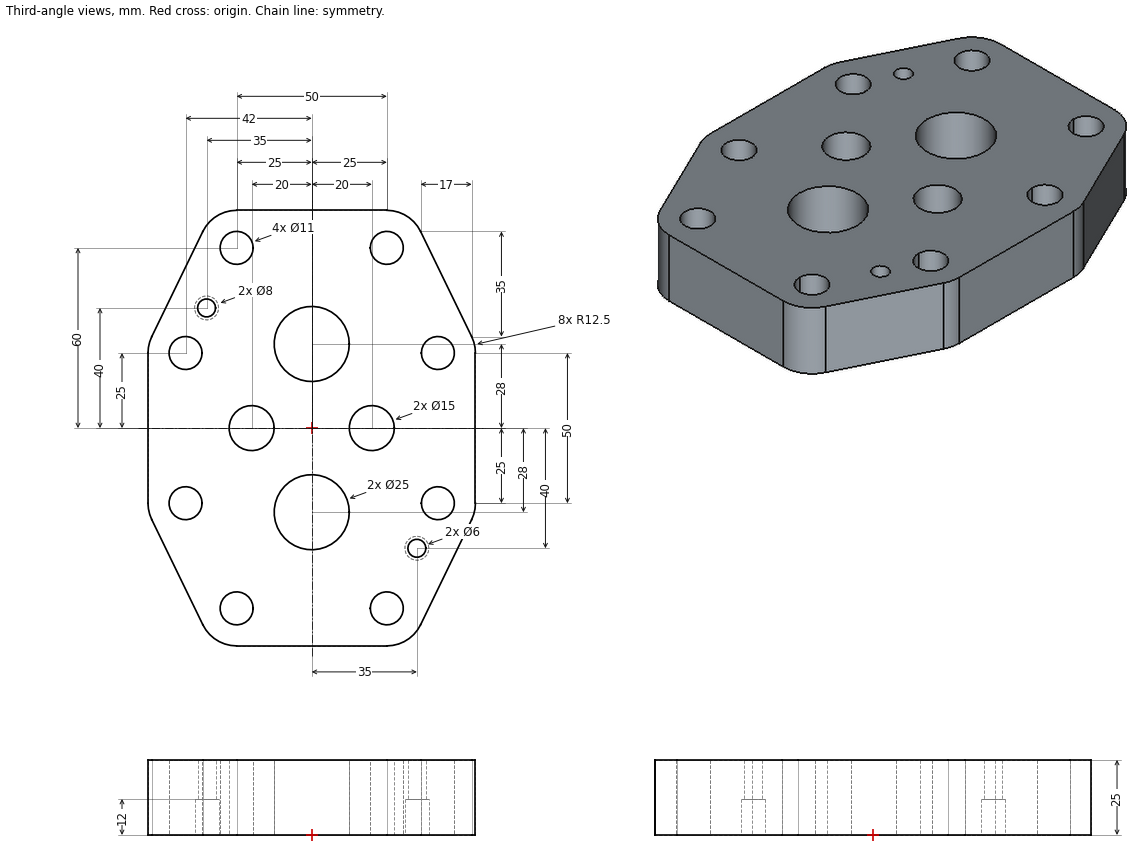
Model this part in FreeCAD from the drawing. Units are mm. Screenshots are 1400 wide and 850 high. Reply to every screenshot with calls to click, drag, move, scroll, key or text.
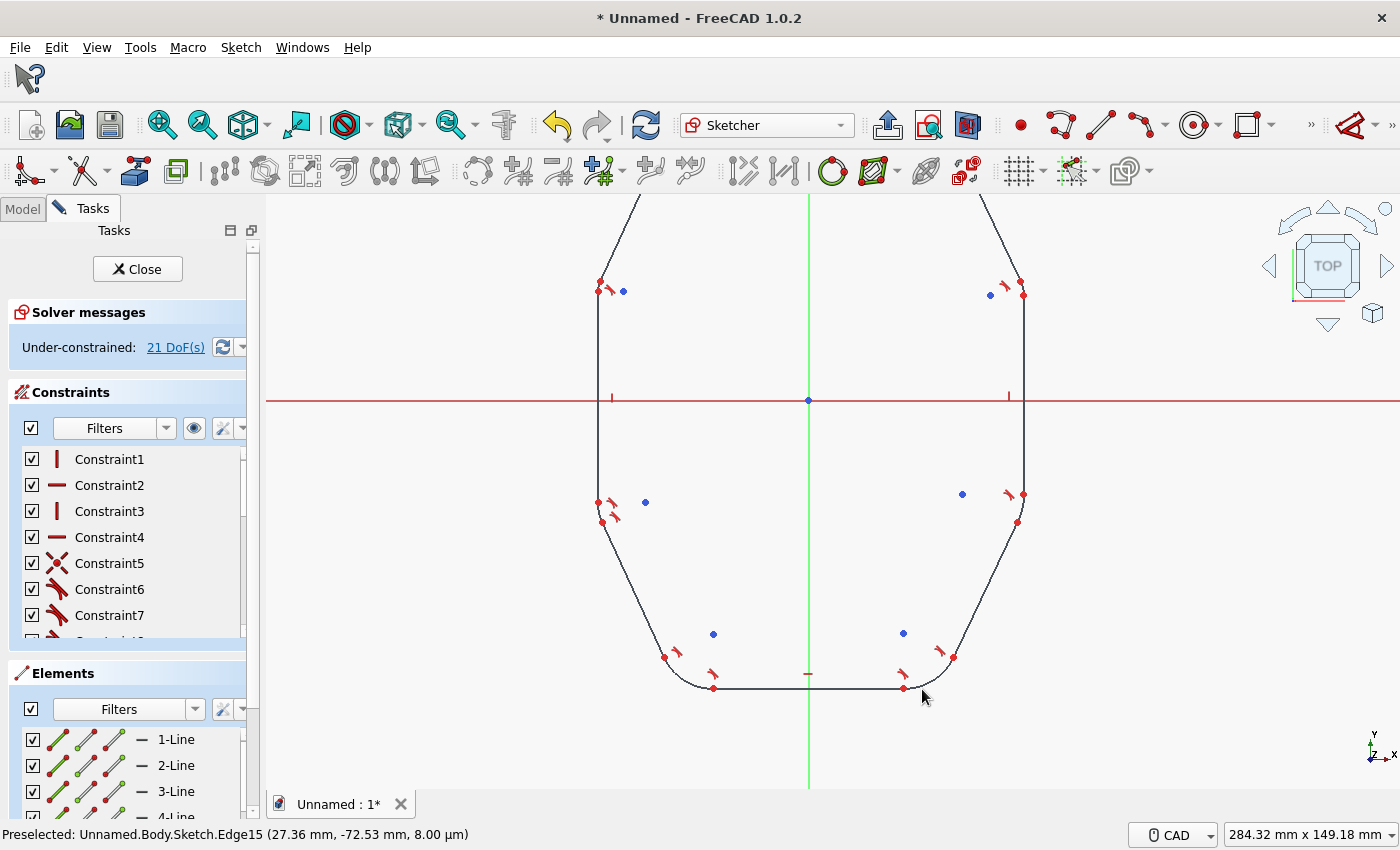
click(973, 617)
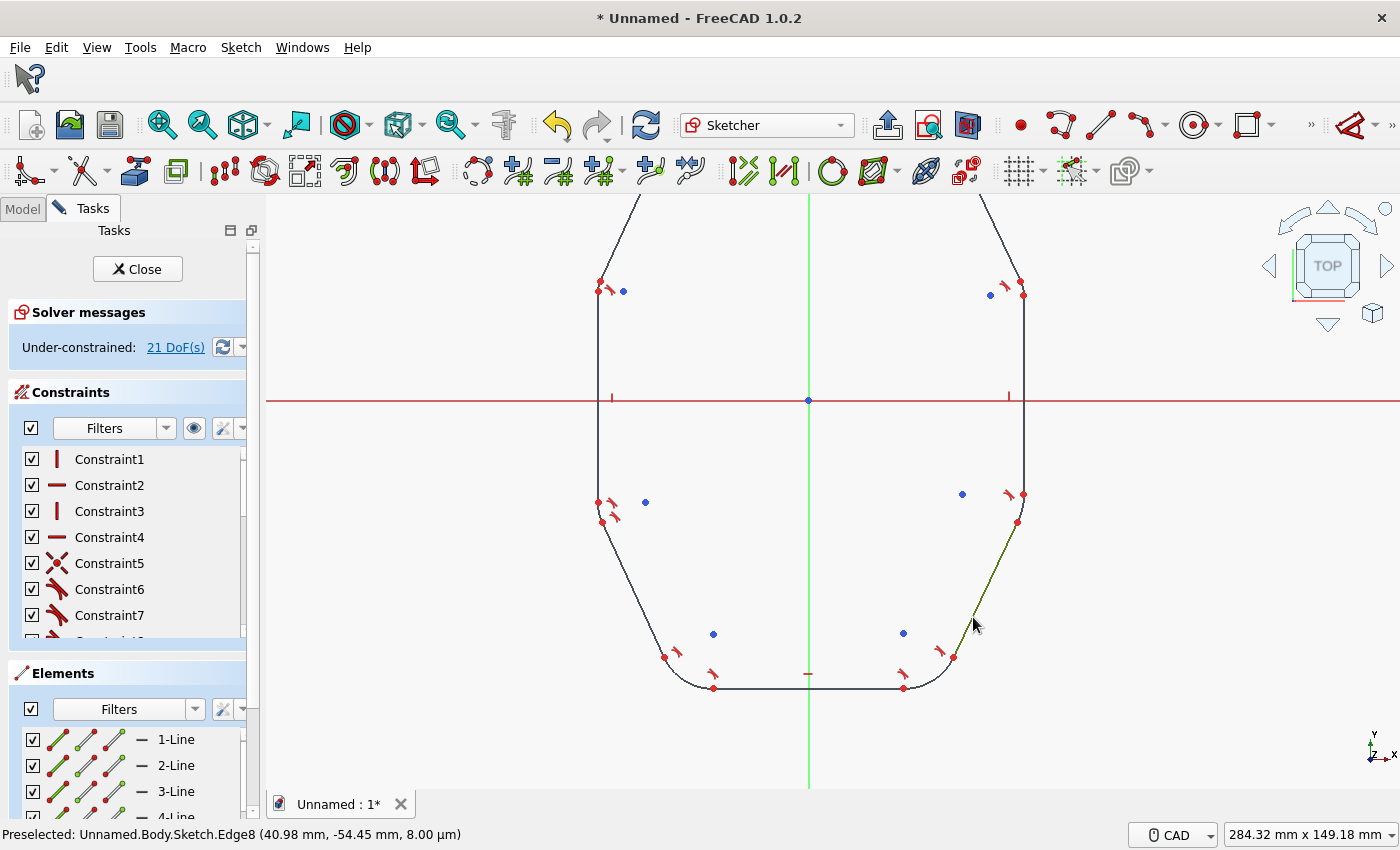
click(1022, 509)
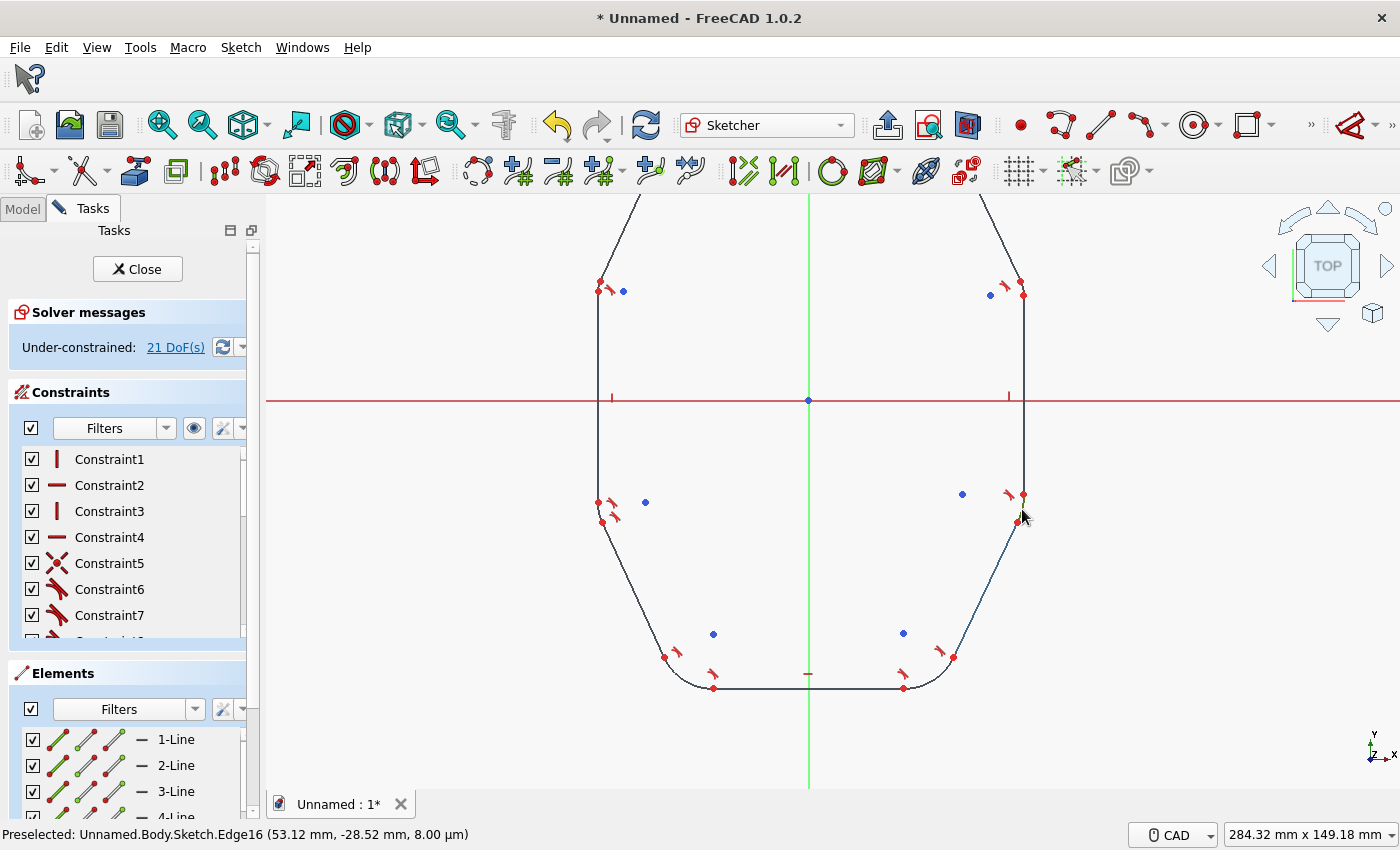
key(t)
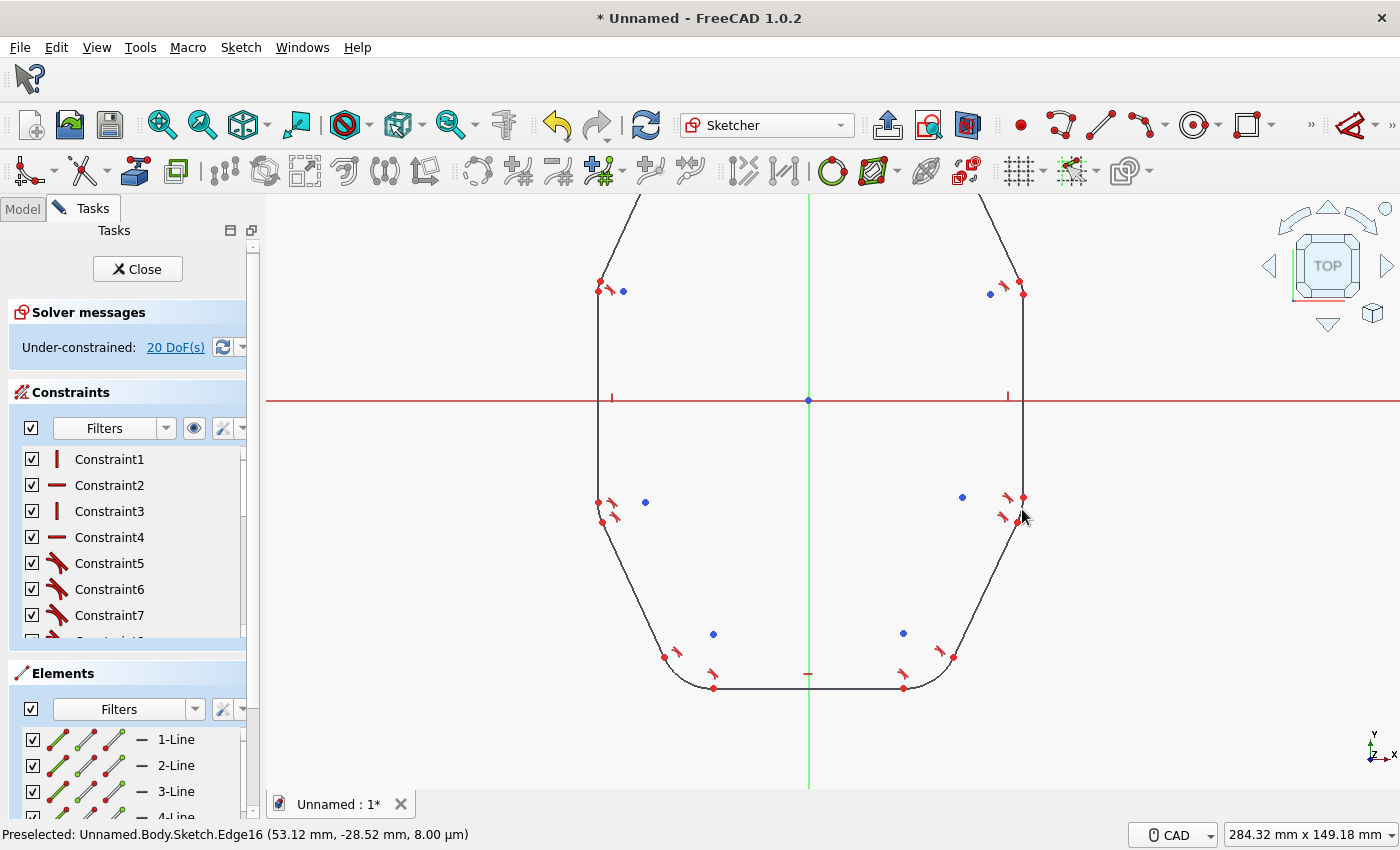
scroll(1022, 288, up, 4)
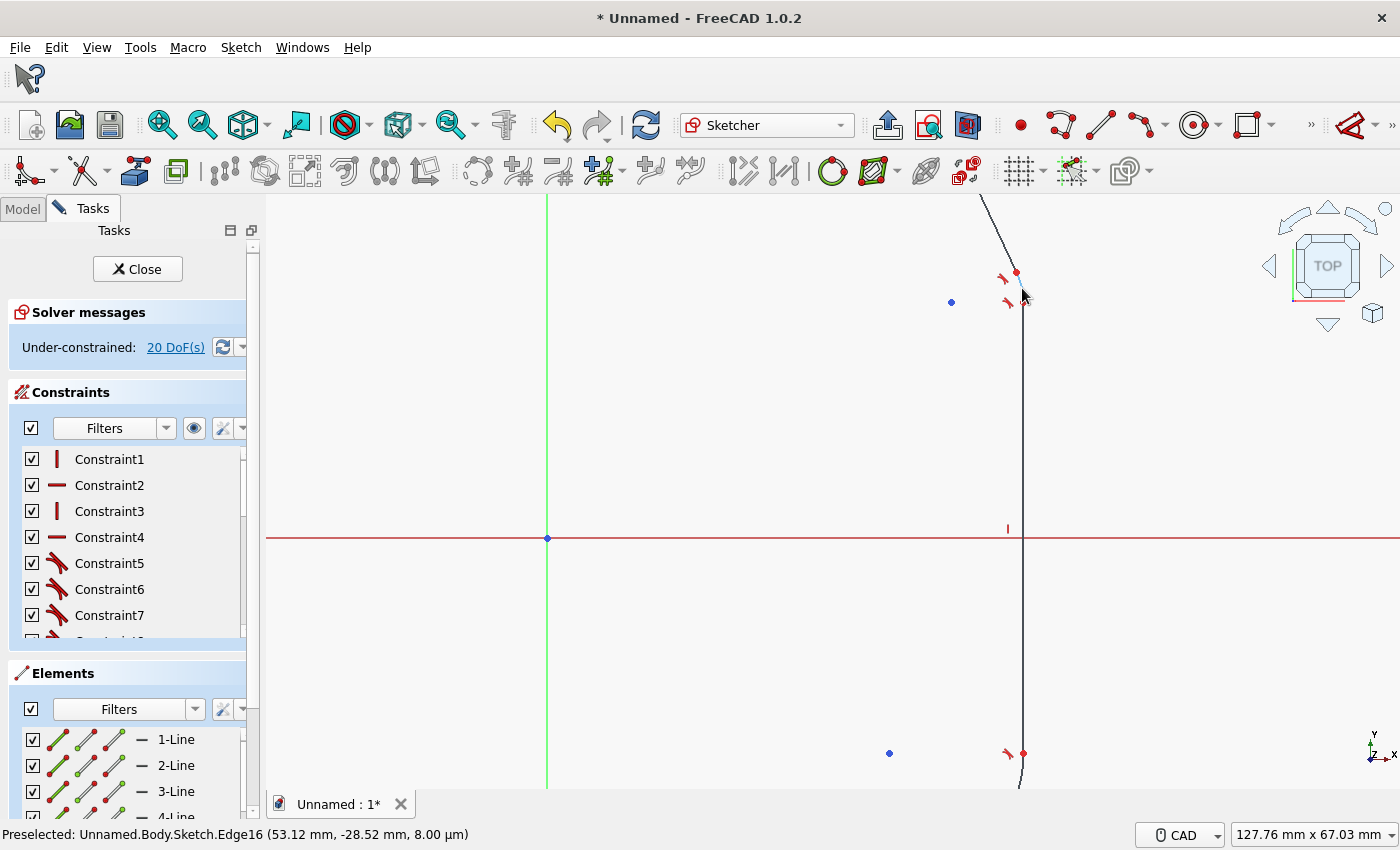
click(1022, 287)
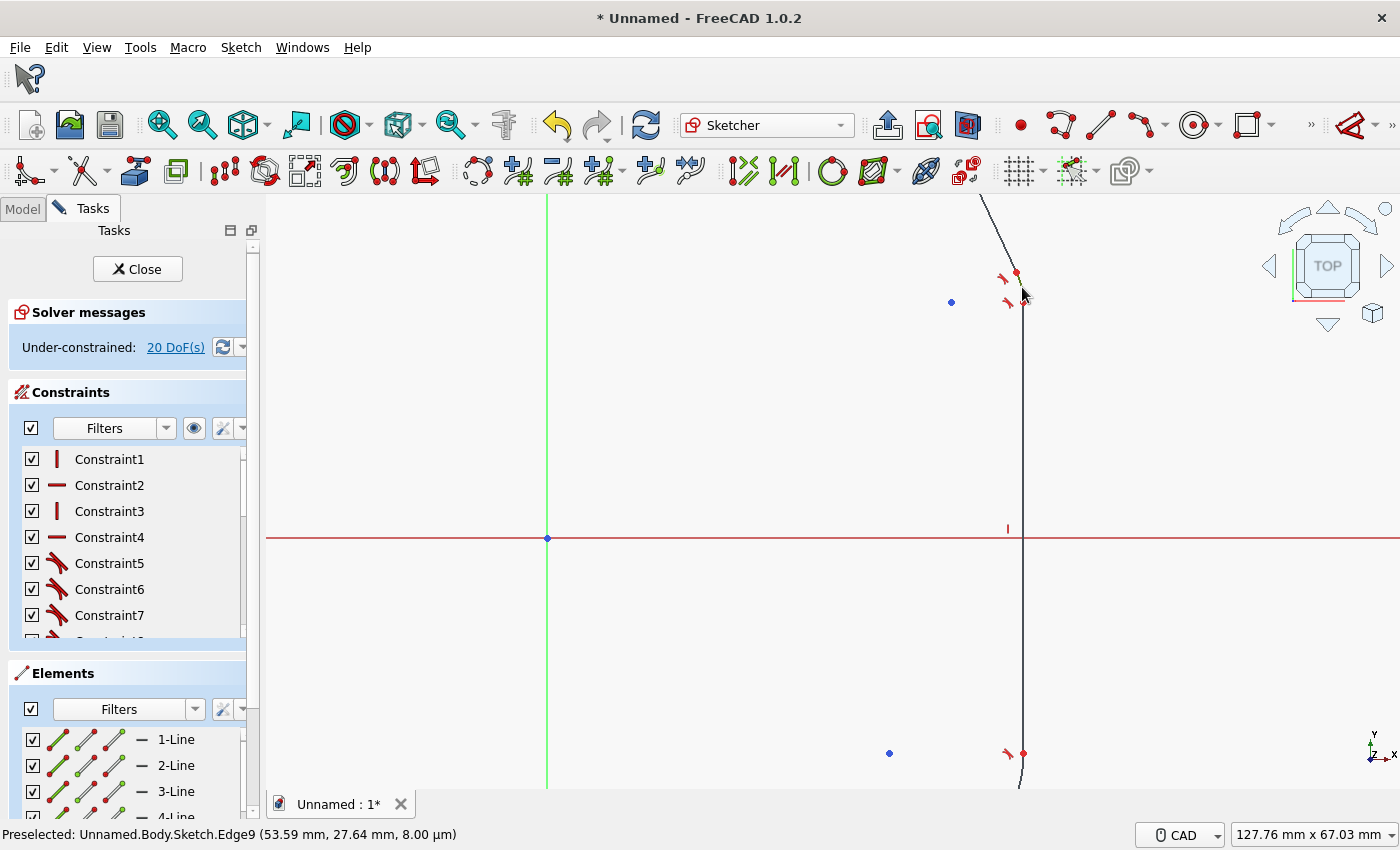
scroll(858, 471, down, 6)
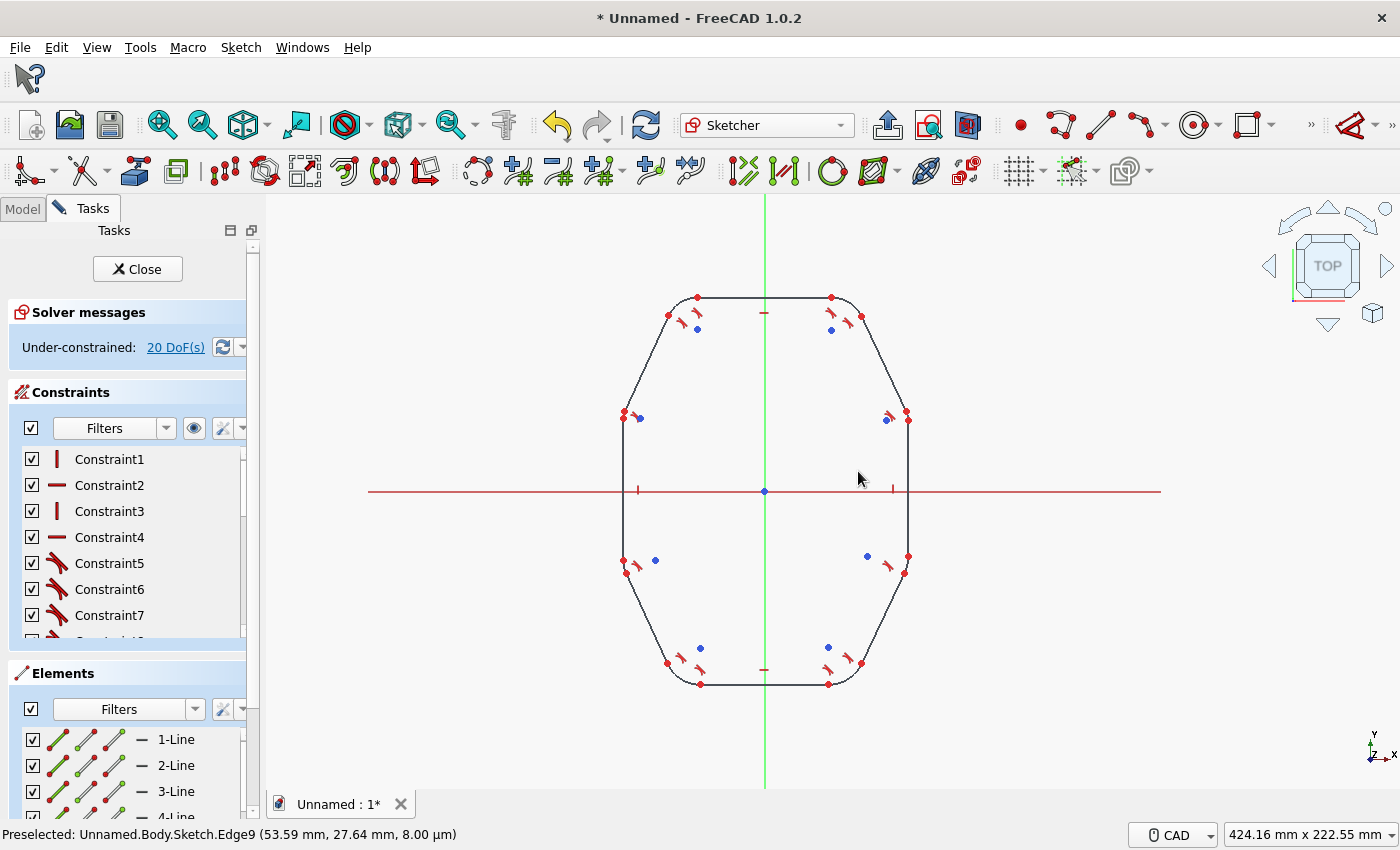
scroll(855, 307, up, 2)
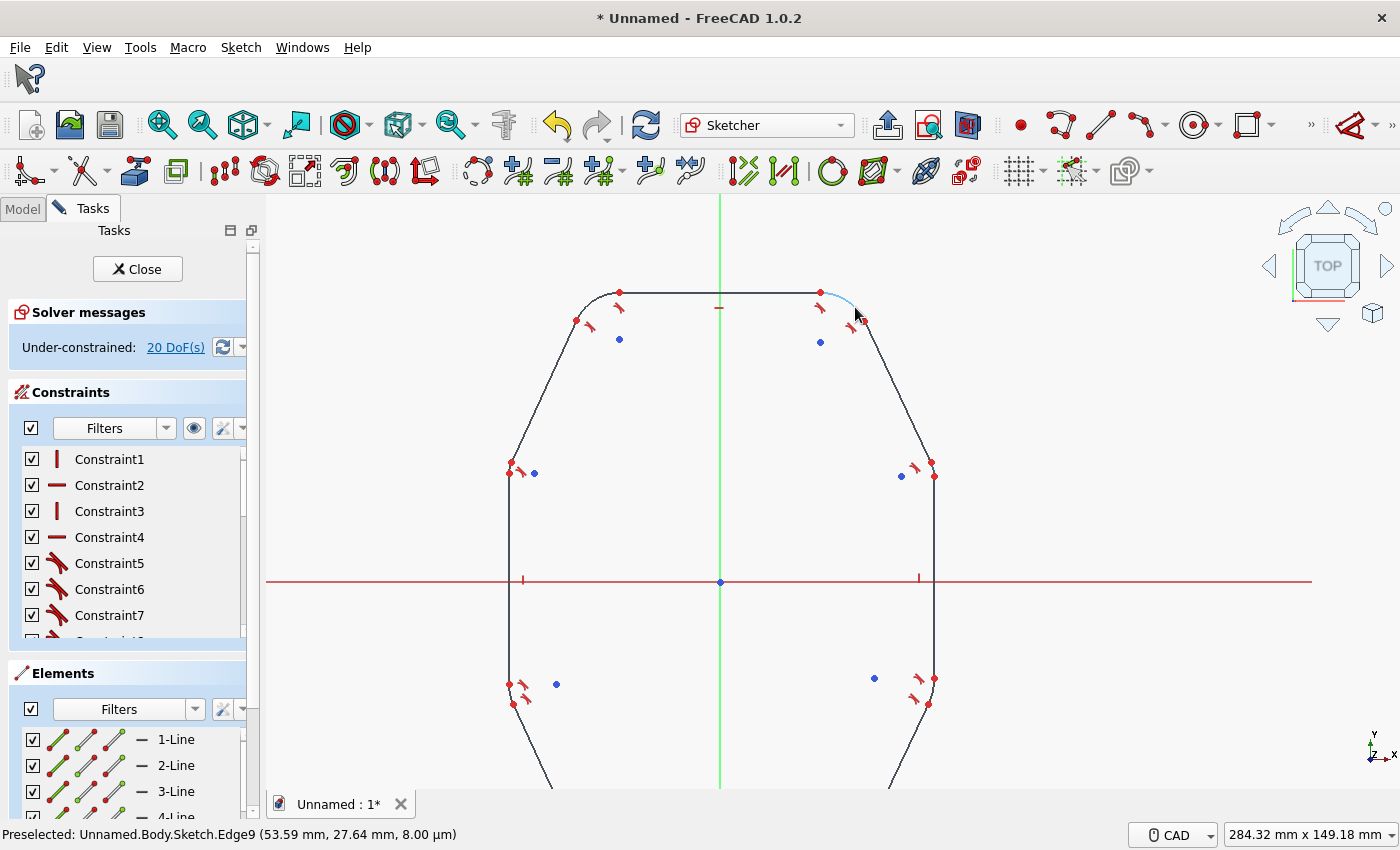
click(855, 308)